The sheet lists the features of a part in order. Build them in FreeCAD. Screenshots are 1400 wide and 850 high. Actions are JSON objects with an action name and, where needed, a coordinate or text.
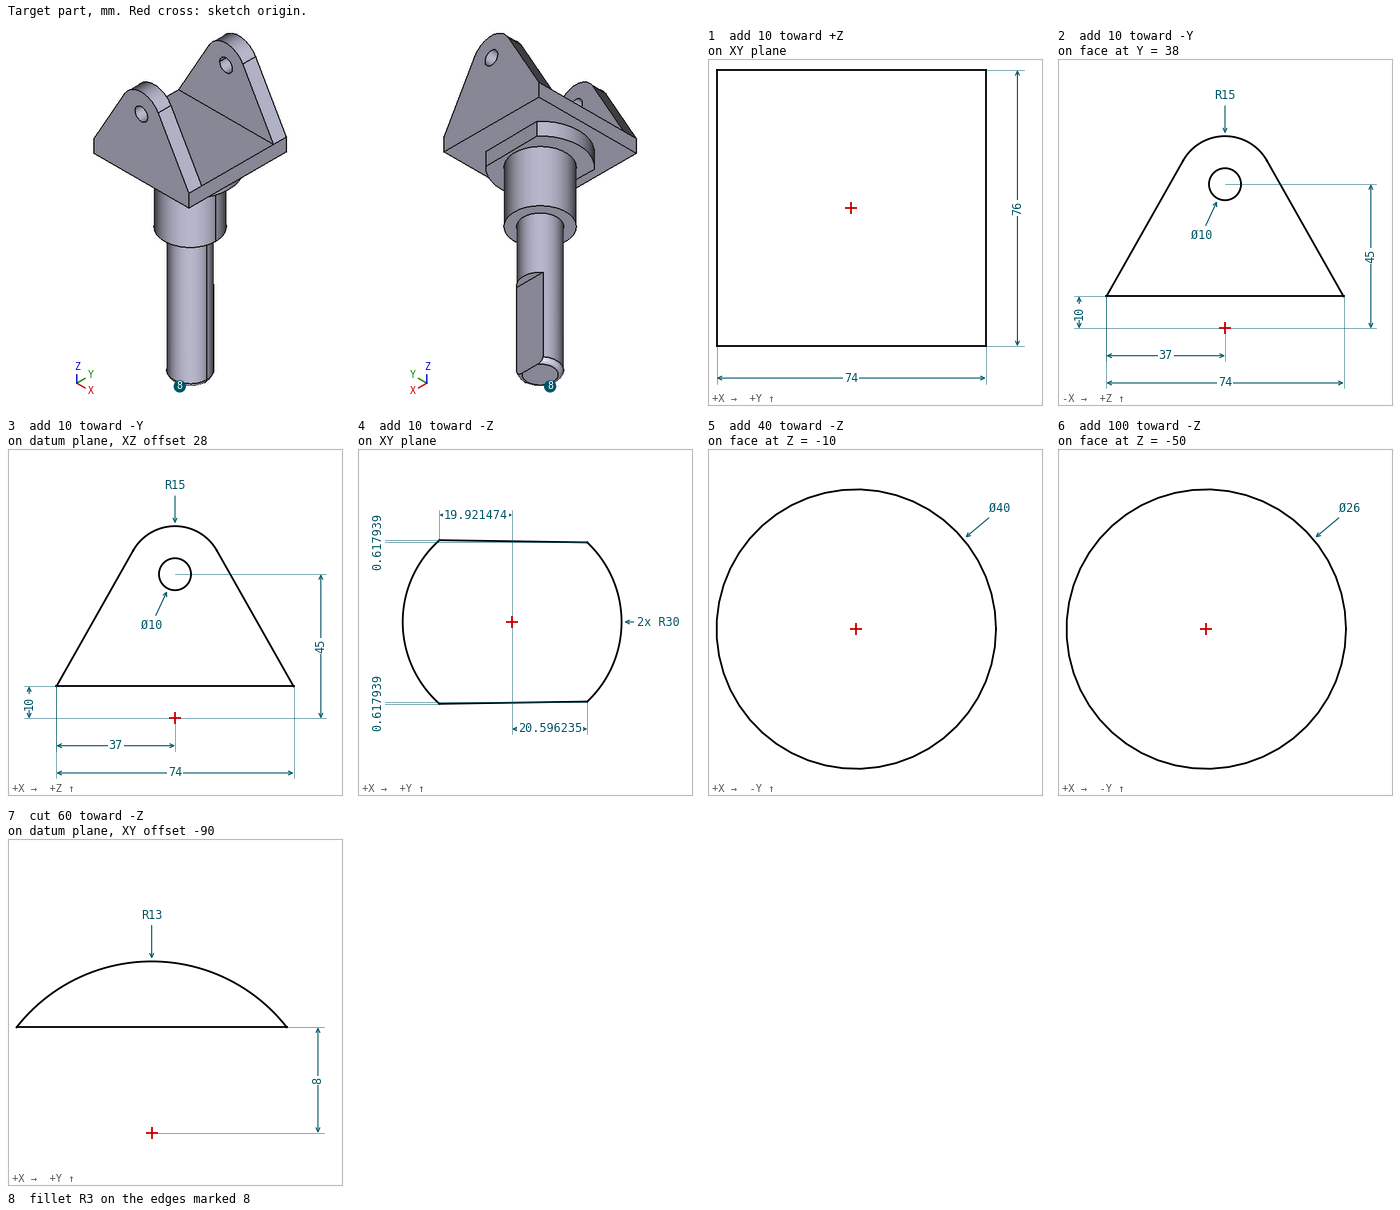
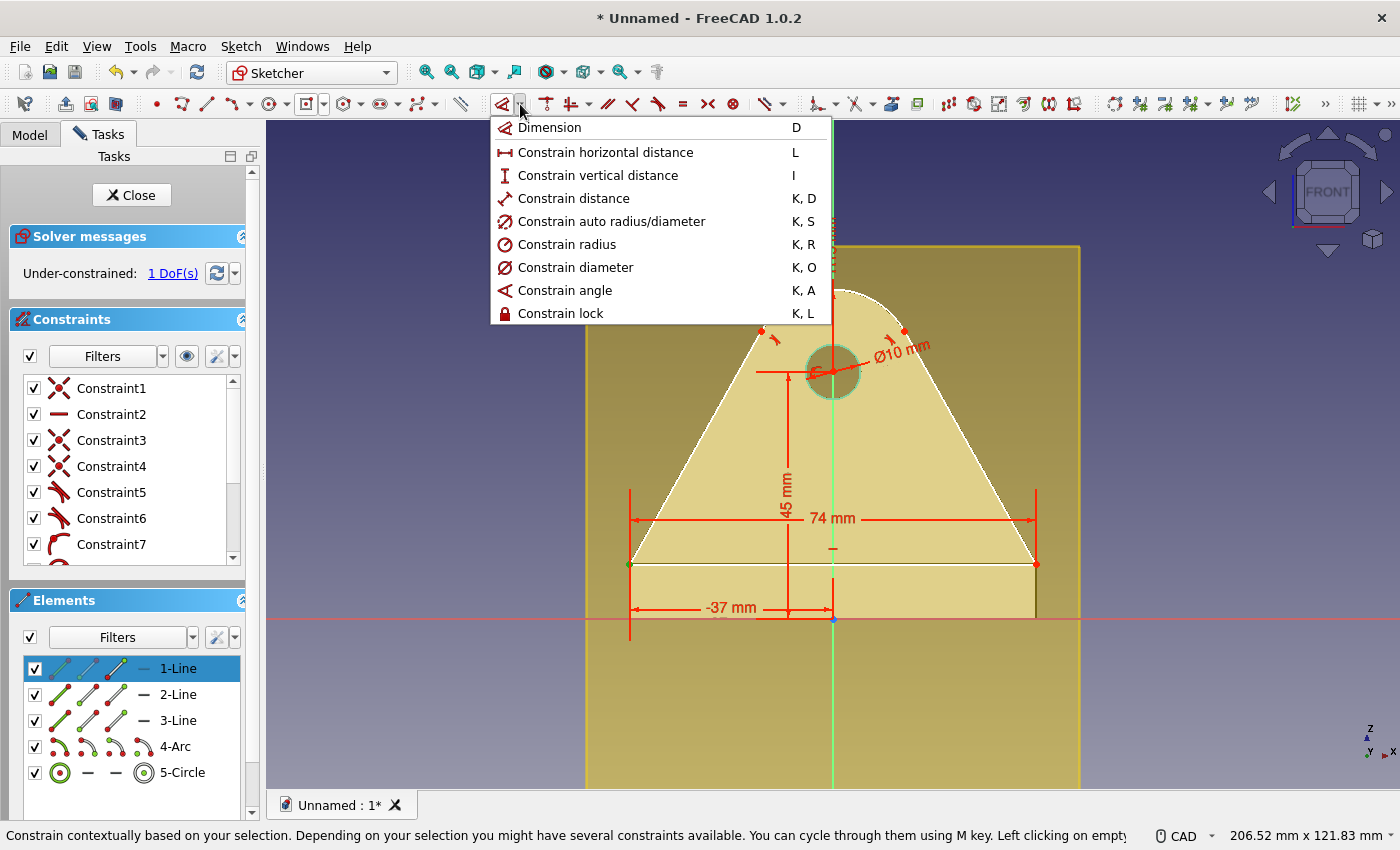
{"action": "left_click", "coordinate": [661, 176]}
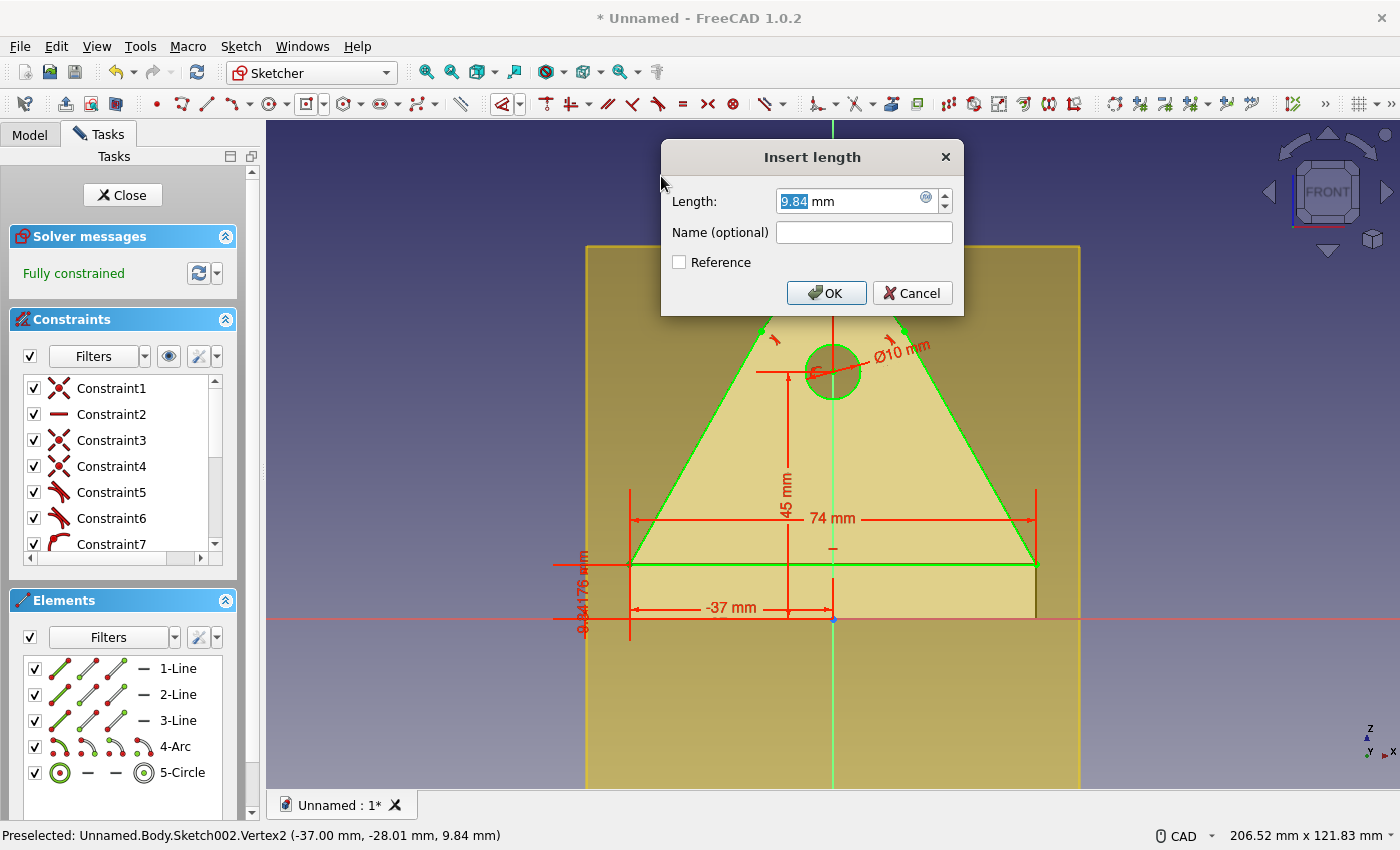
{"action": "type", "text": "10"}
{"action": "key", "text": "Return"}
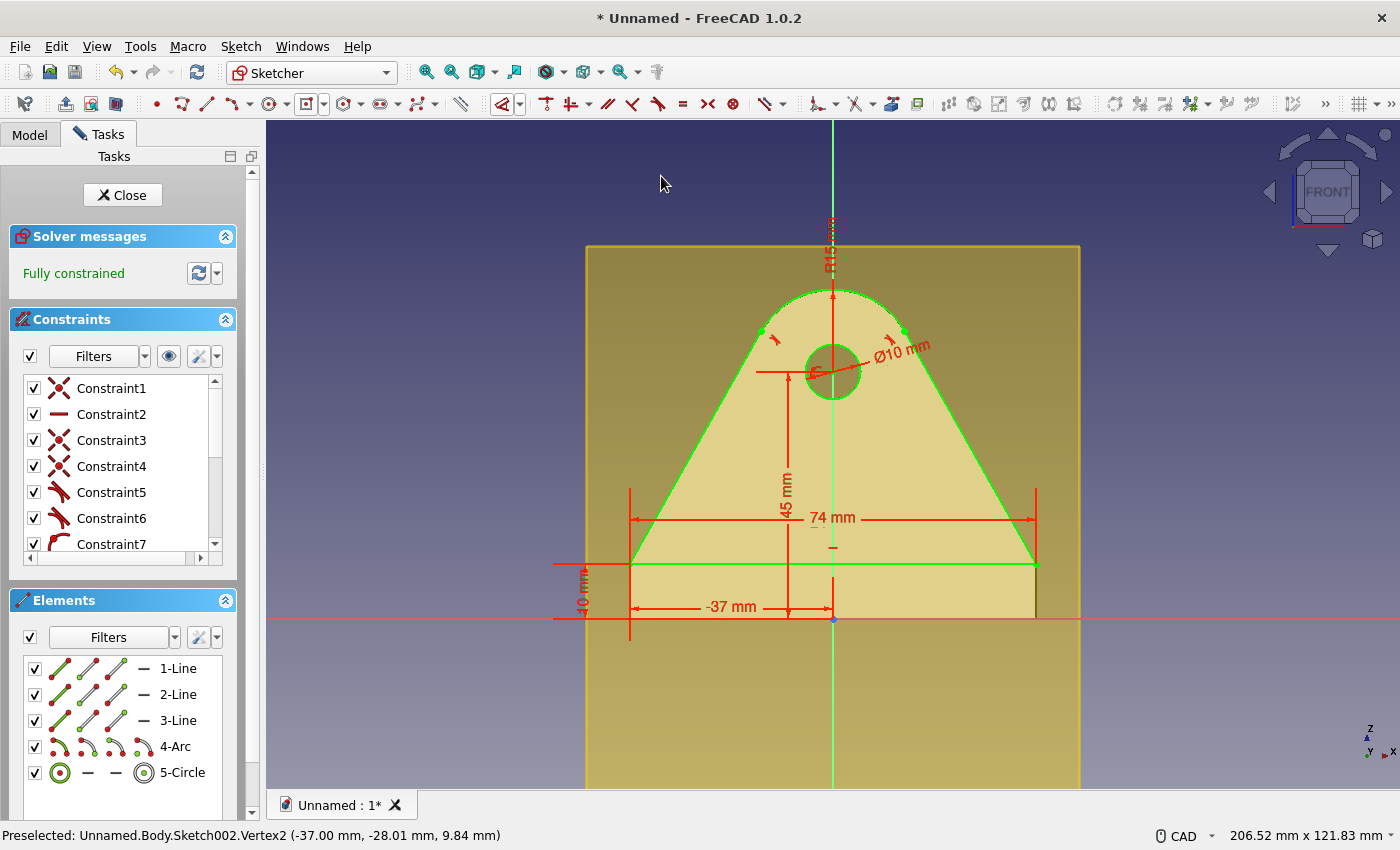
{"action": "left_click", "coordinate": [123, 195]}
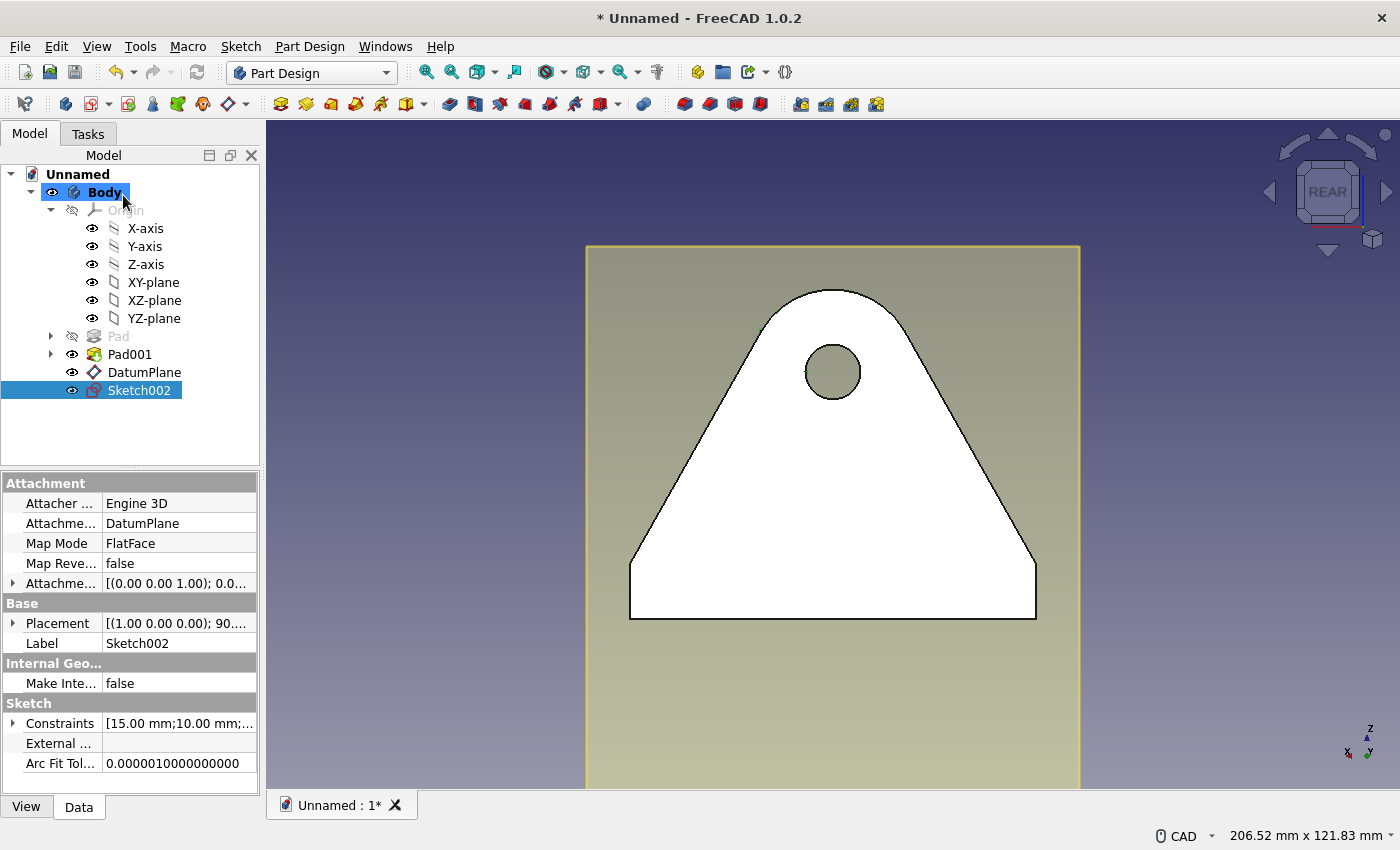
{"action": "left_click", "coordinate": [281, 104]}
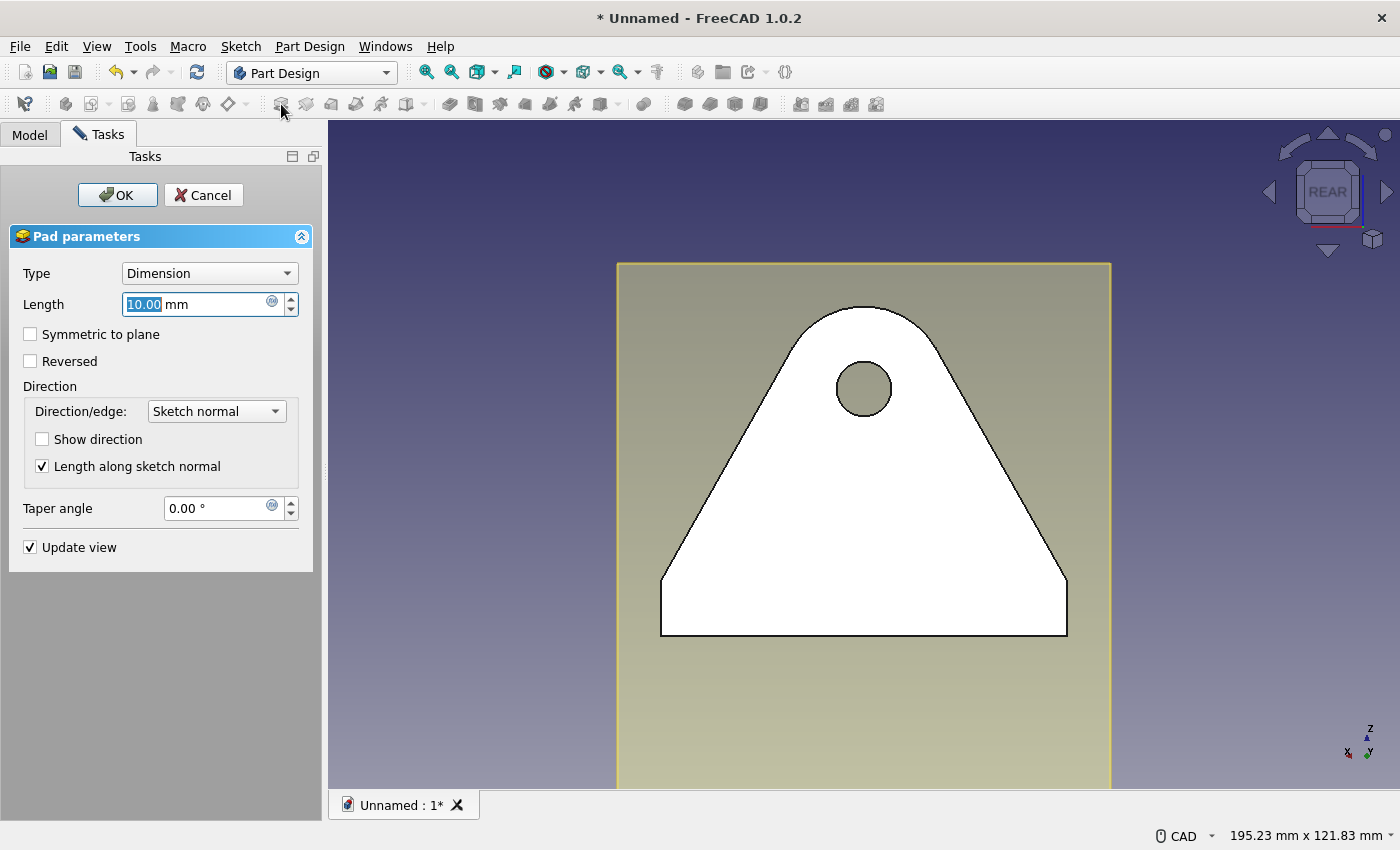
{"action": "type", "text": "10"}
{"action": "key", "text": "Tab"}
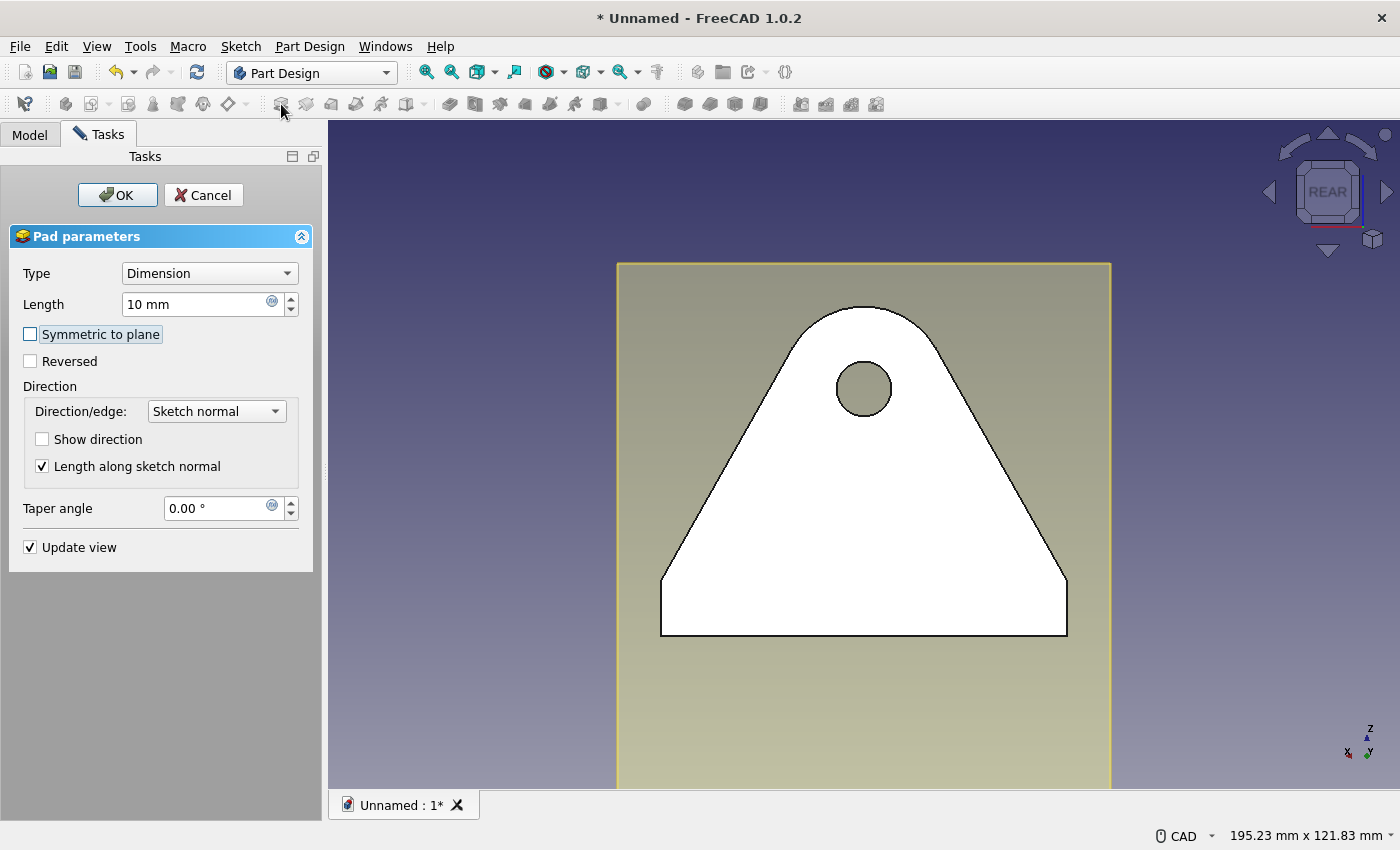
{"action": "left_click", "coordinate": [118, 195]}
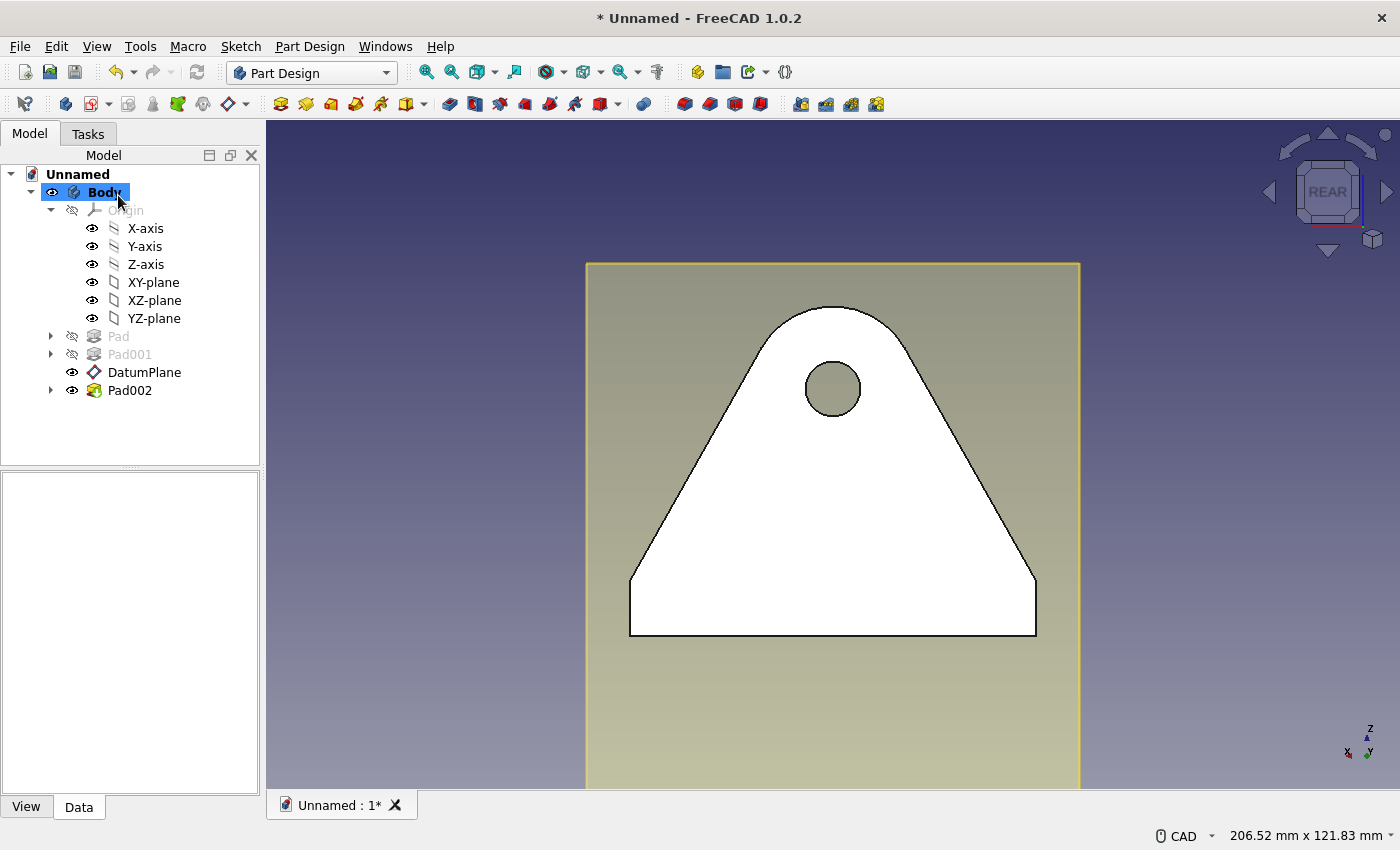
{"action": "left_click", "coordinate": [117, 372]}
{"action": "key", "text": "space"}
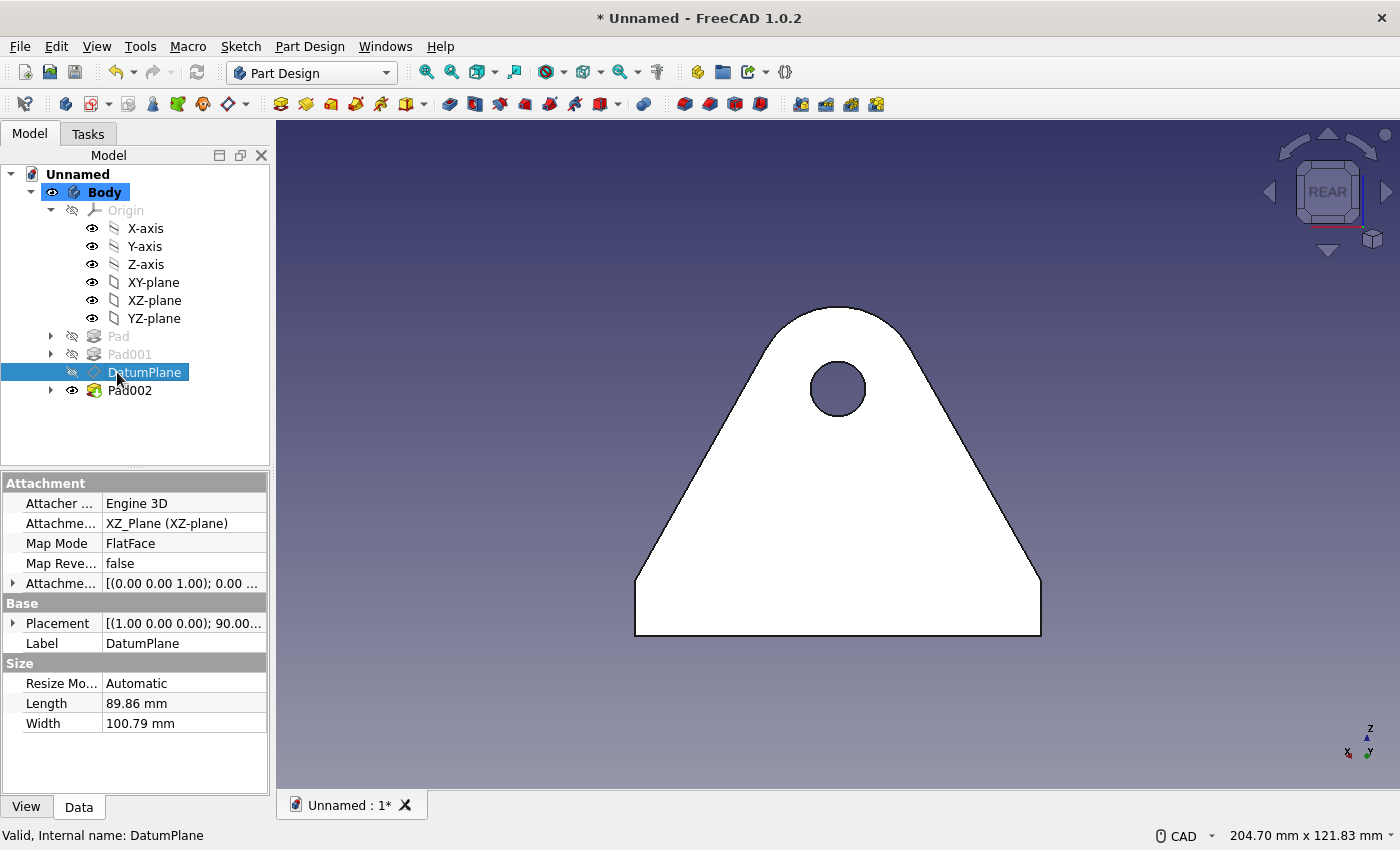
{"action": "left_click", "coordinate": [316, 749]}